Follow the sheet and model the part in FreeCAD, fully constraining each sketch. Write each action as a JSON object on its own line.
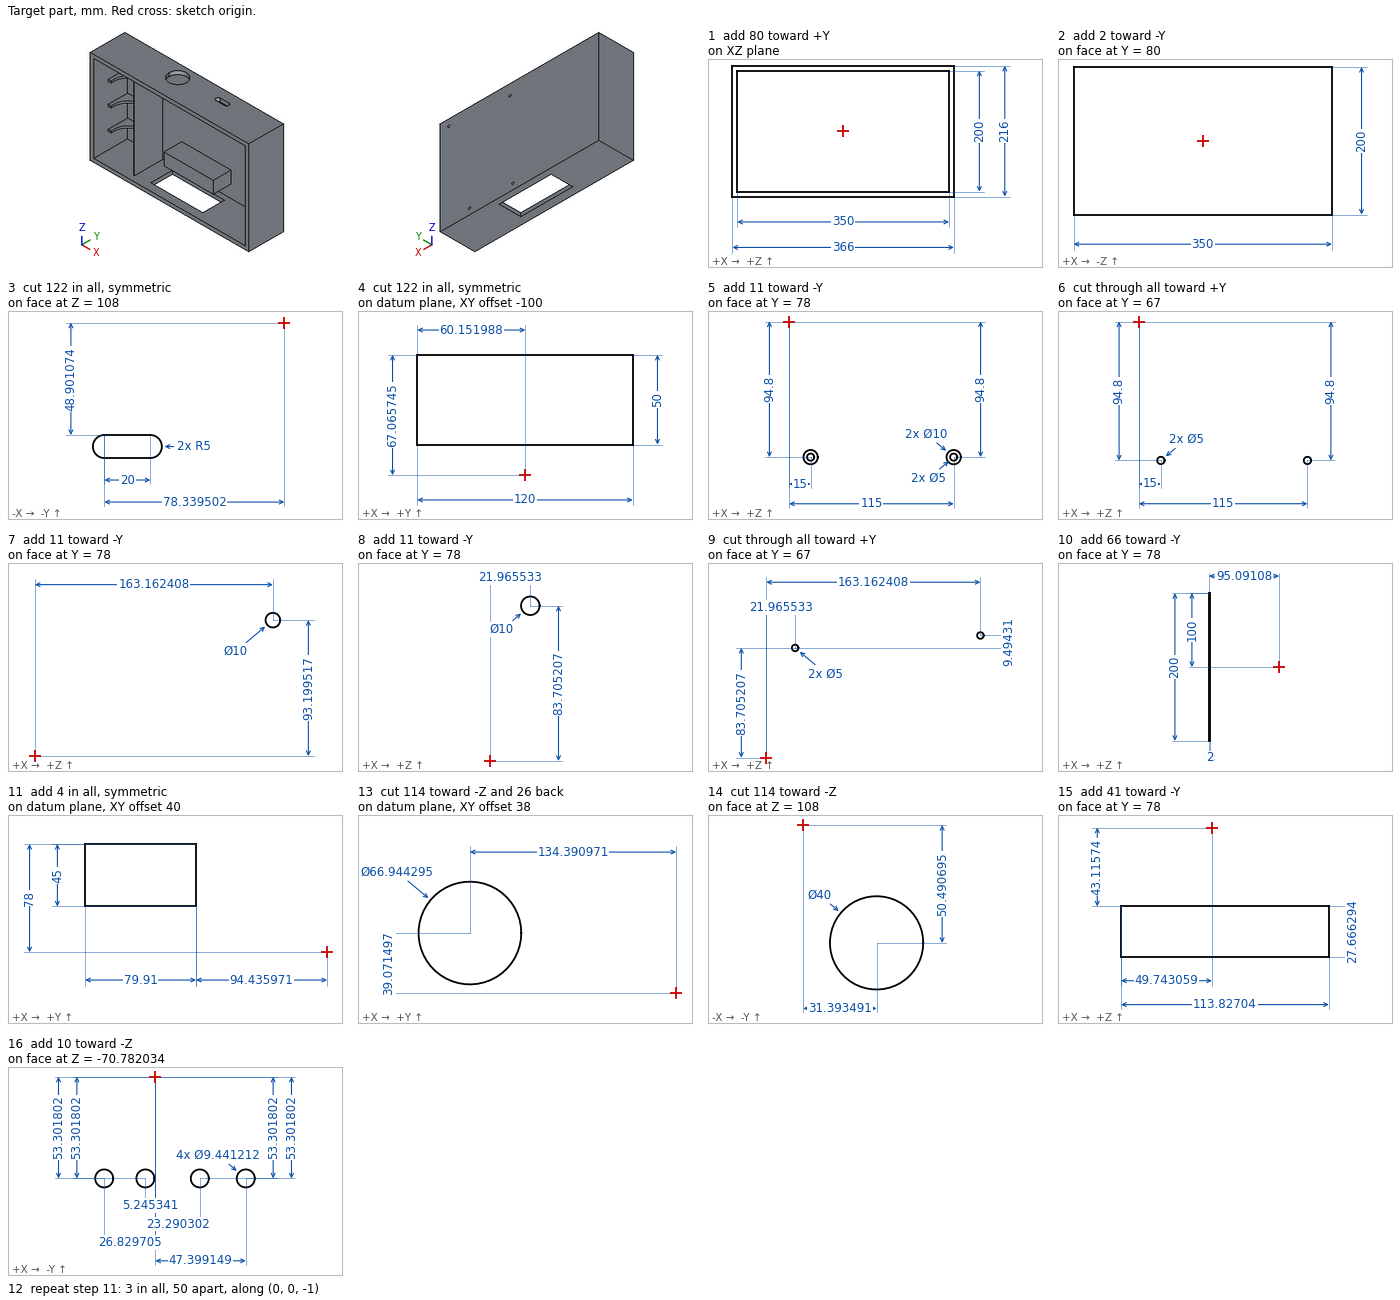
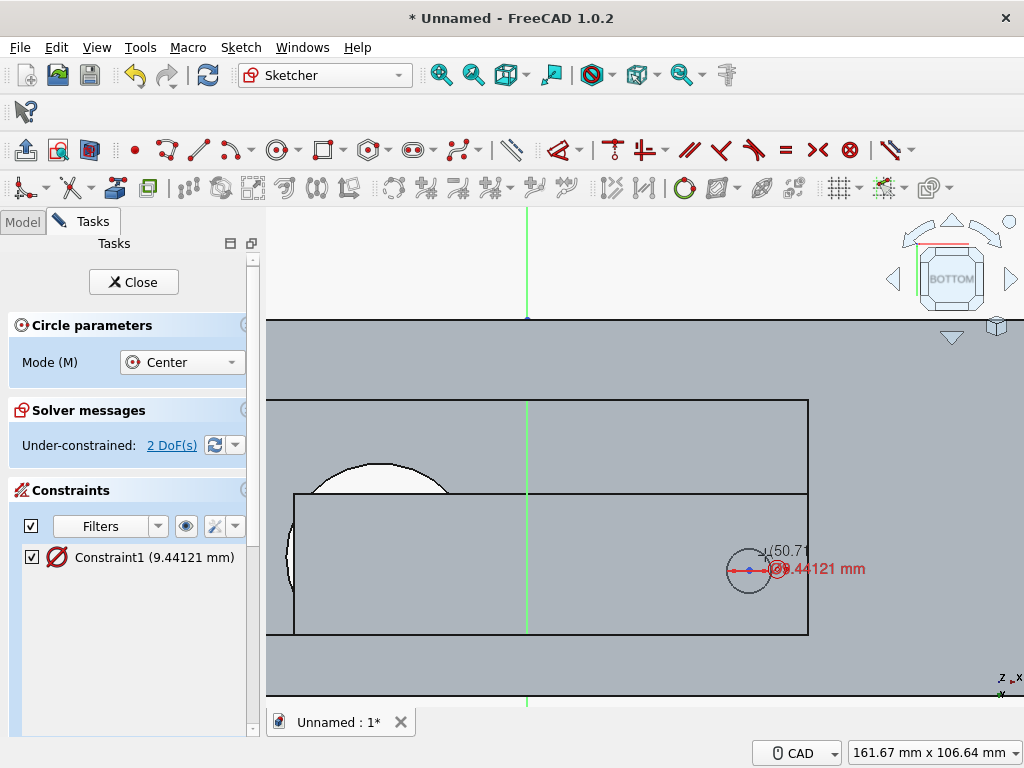
{"action": "left_click", "coordinate": [636, 570]}
{"action": "mouse_move", "coordinate": [652, 555]}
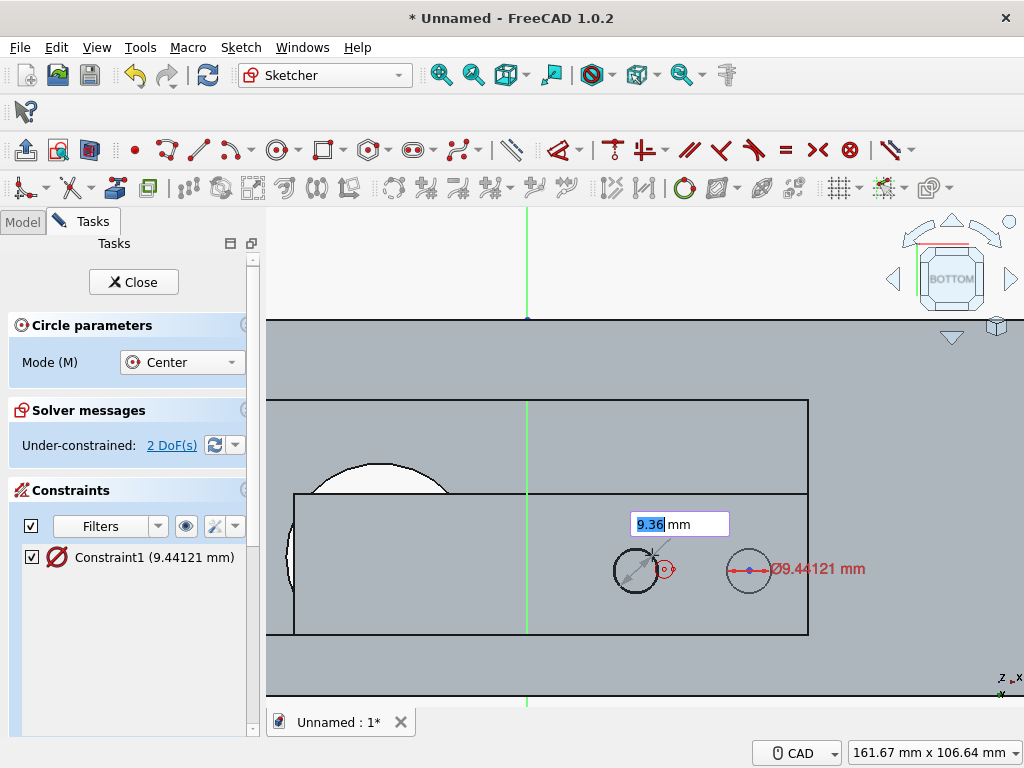
{"action": "type", "text": "9.441212"}
{"action": "key", "text": "Return"}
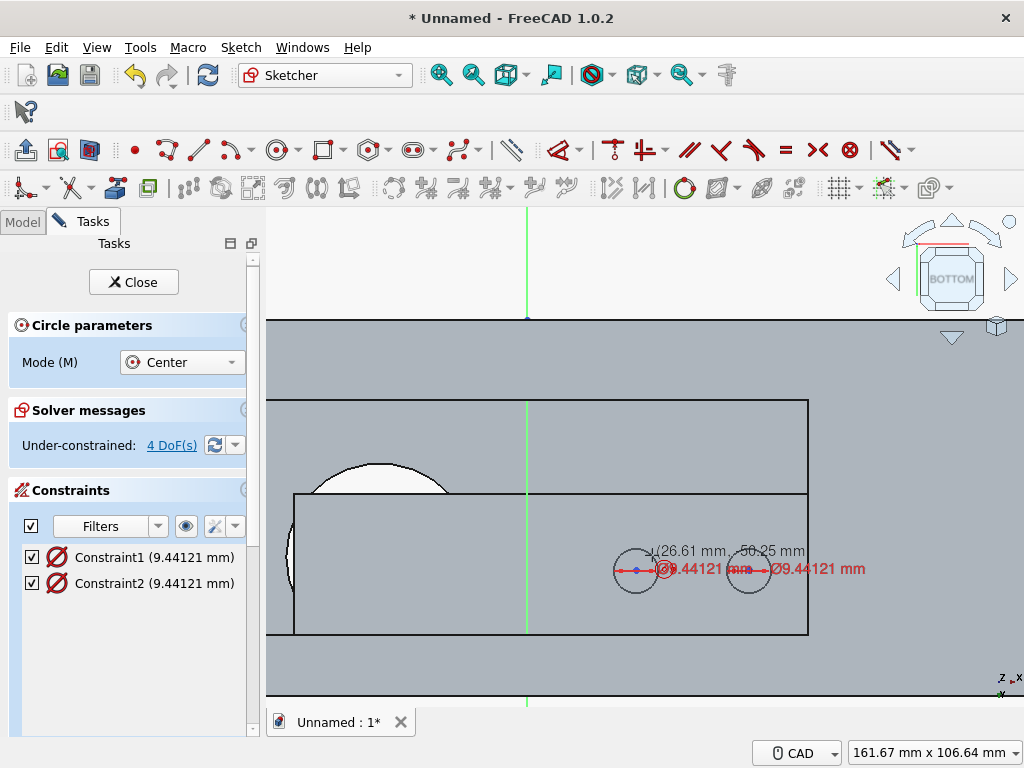
{"action": "left_click", "coordinate": [503, 570]}
{"action": "mouse_move", "coordinate": [487, 555]}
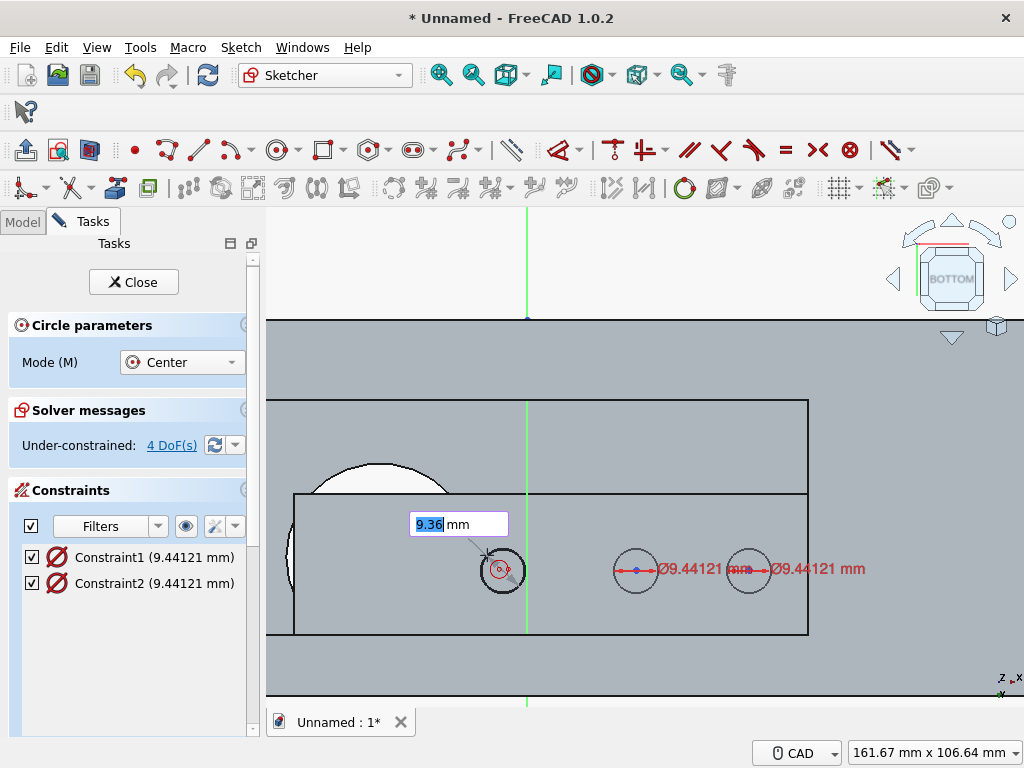
{"action": "type", "text": "9.441212"}
{"action": "key", "text": "Return"}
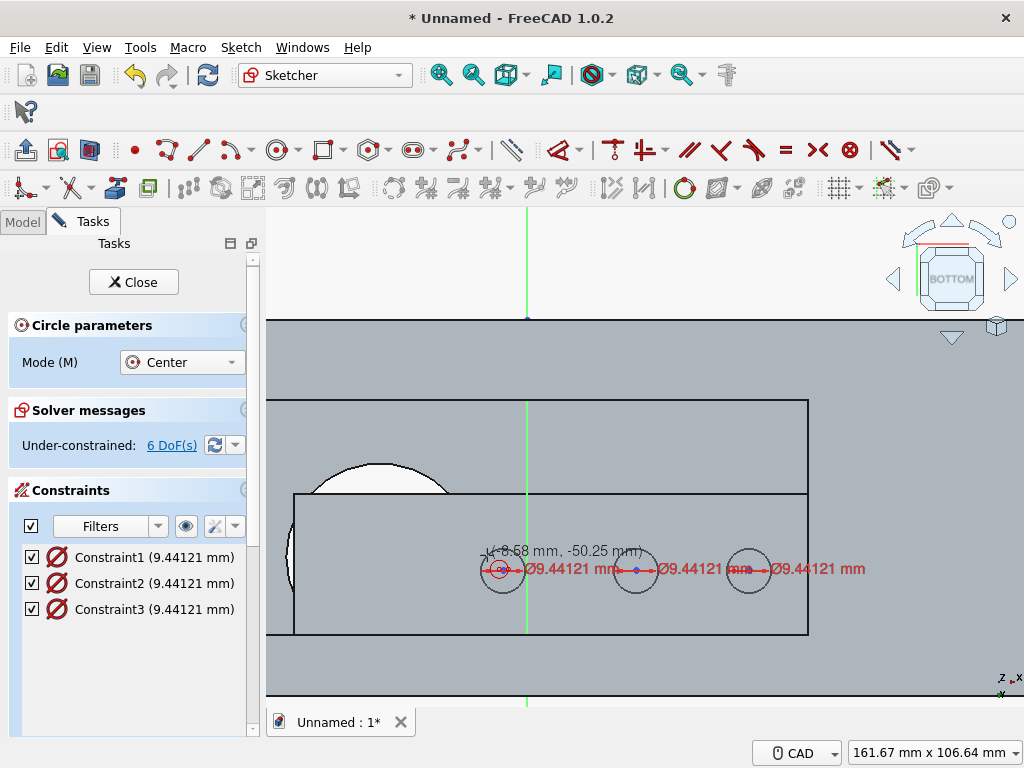
{"action": "left_click", "coordinate": [401, 570]}
{"action": "mouse_move", "coordinate": [417, 555]}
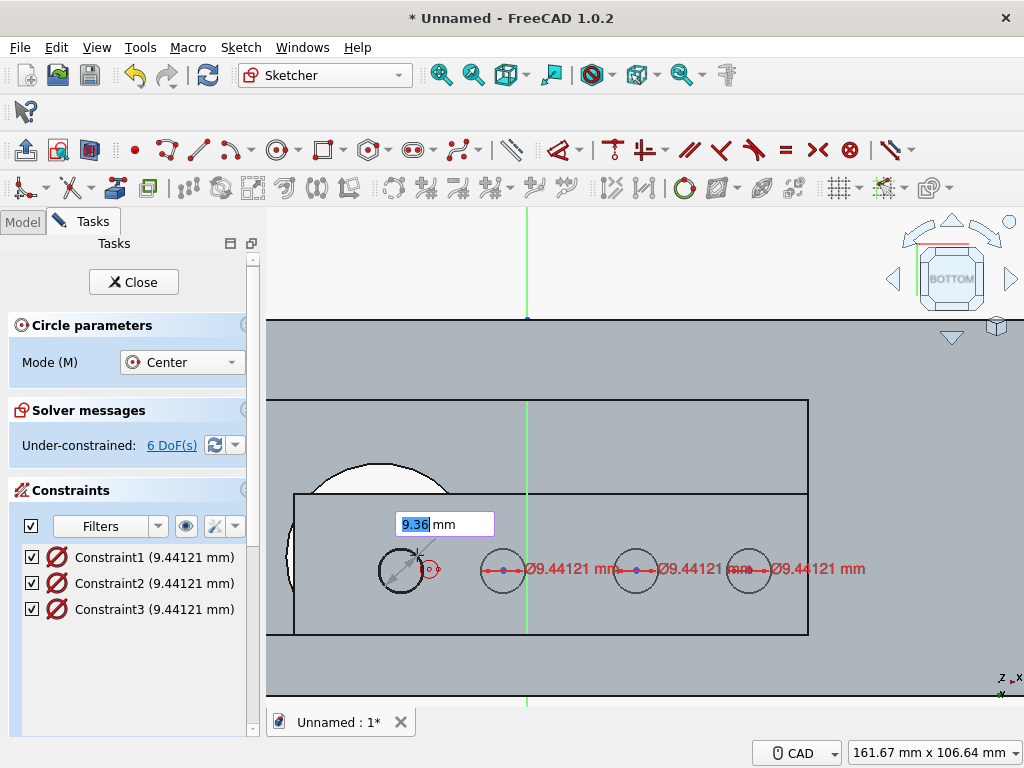
{"action": "type", "text": "9.441212"}
{"action": "key", "text": "Return"}
{"action": "key", "text": "Escape"}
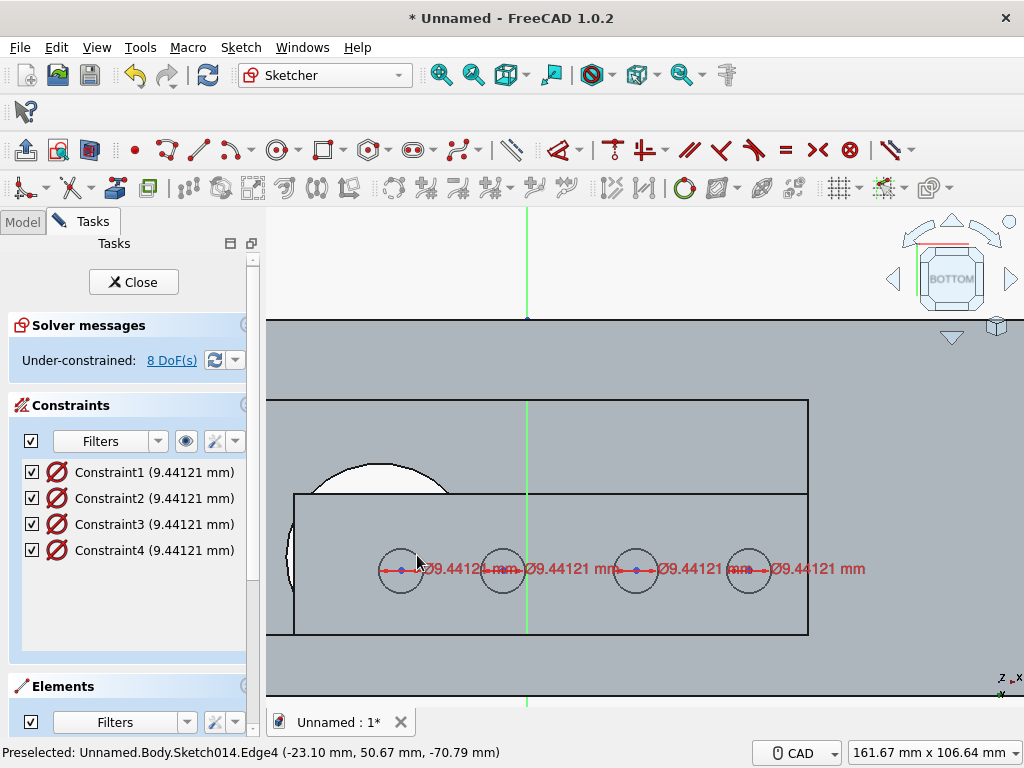
{"action": "key", "text": "d"}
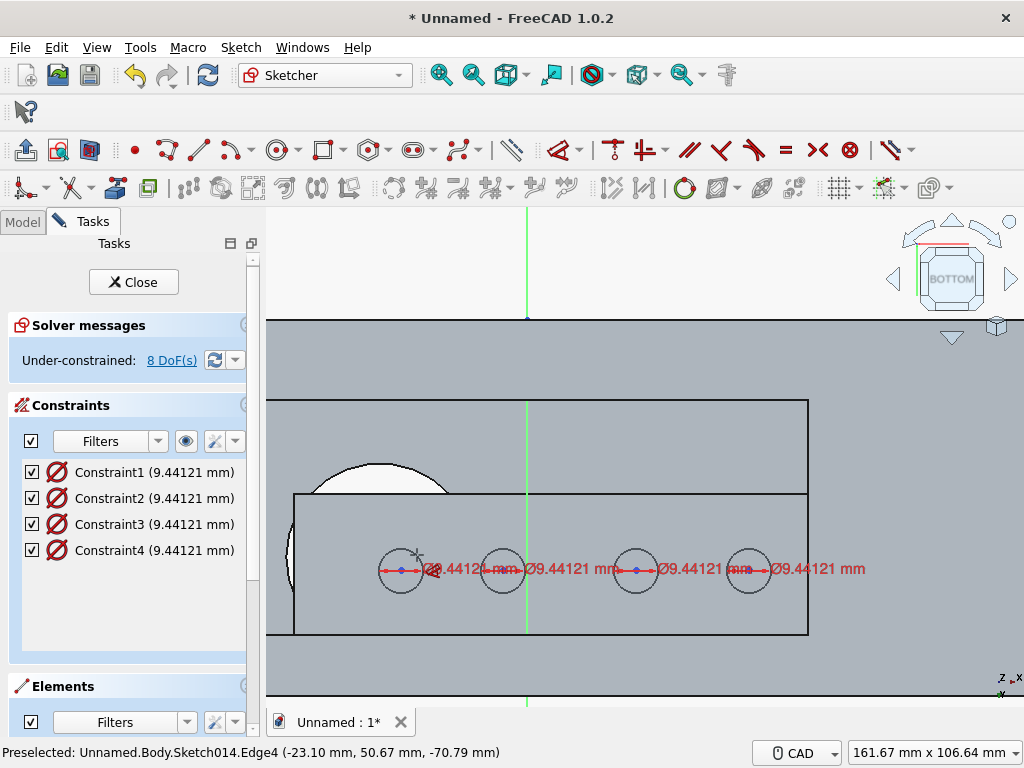
{"action": "scroll", "coordinate": [503, 571], "scroll_direction": "up", "scroll_amount": 3}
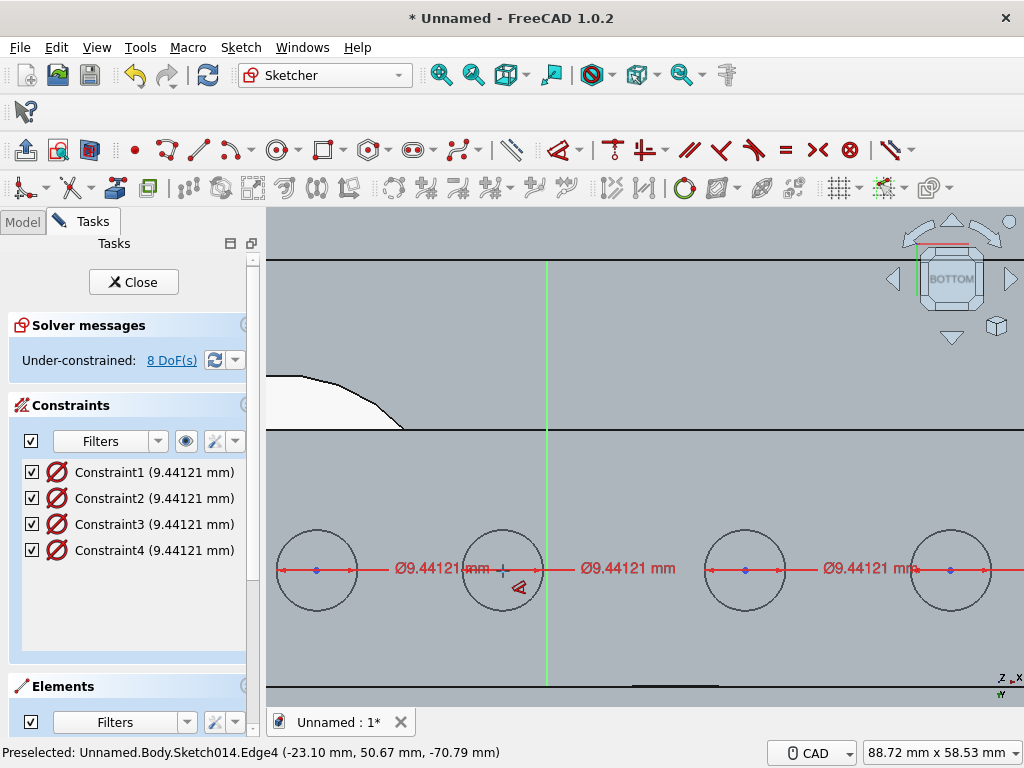
{"action": "left_click", "coordinate": [503, 570]}
{"action": "left_click", "coordinate": [525, 628]}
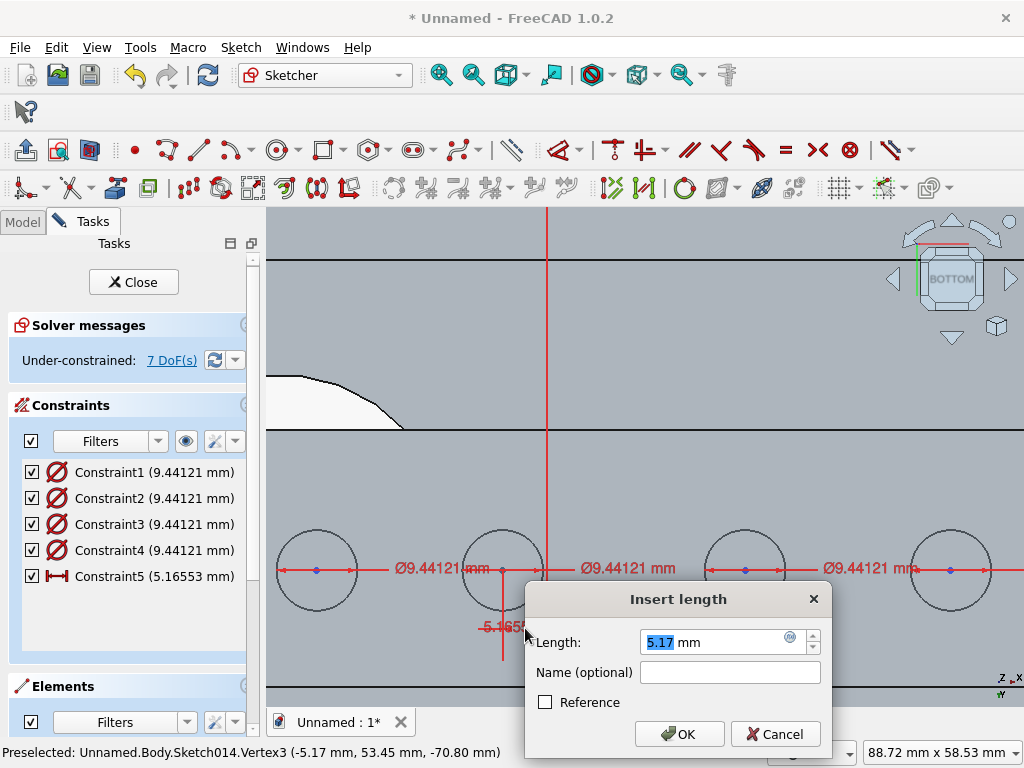
{"action": "type", "text": "5.245341"}
{"action": "key", "text": "Return"}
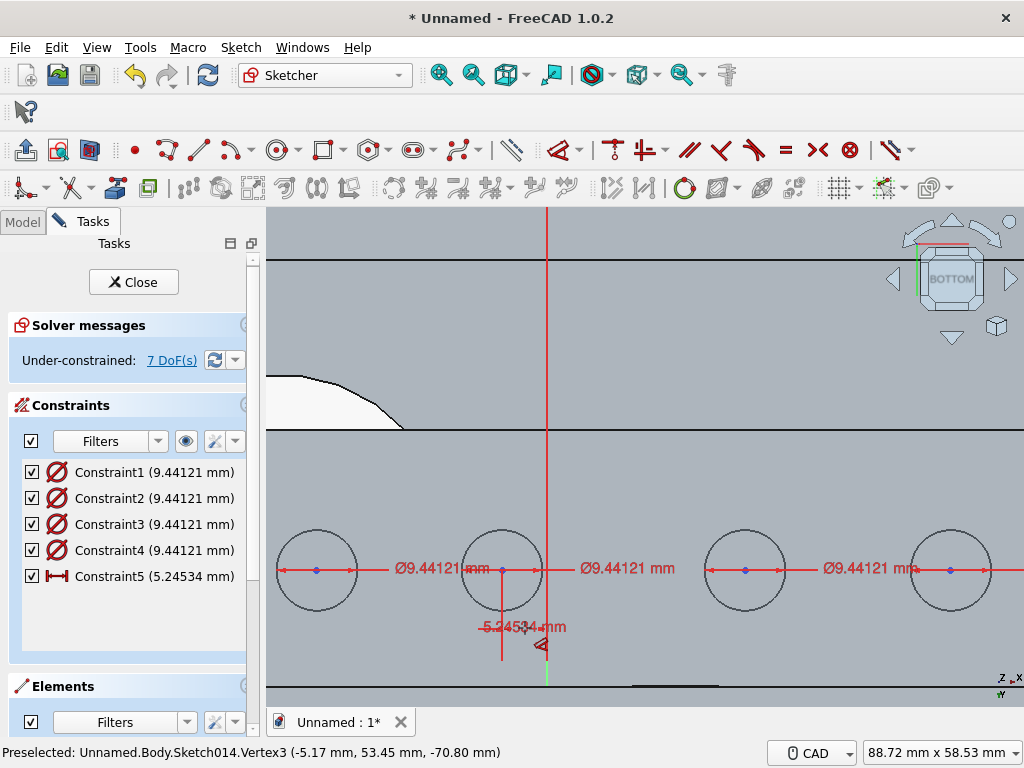
{"action": "scroll", "coordinate": [506, 573], "scroll_direction": "down", "scroll_amount": 3}